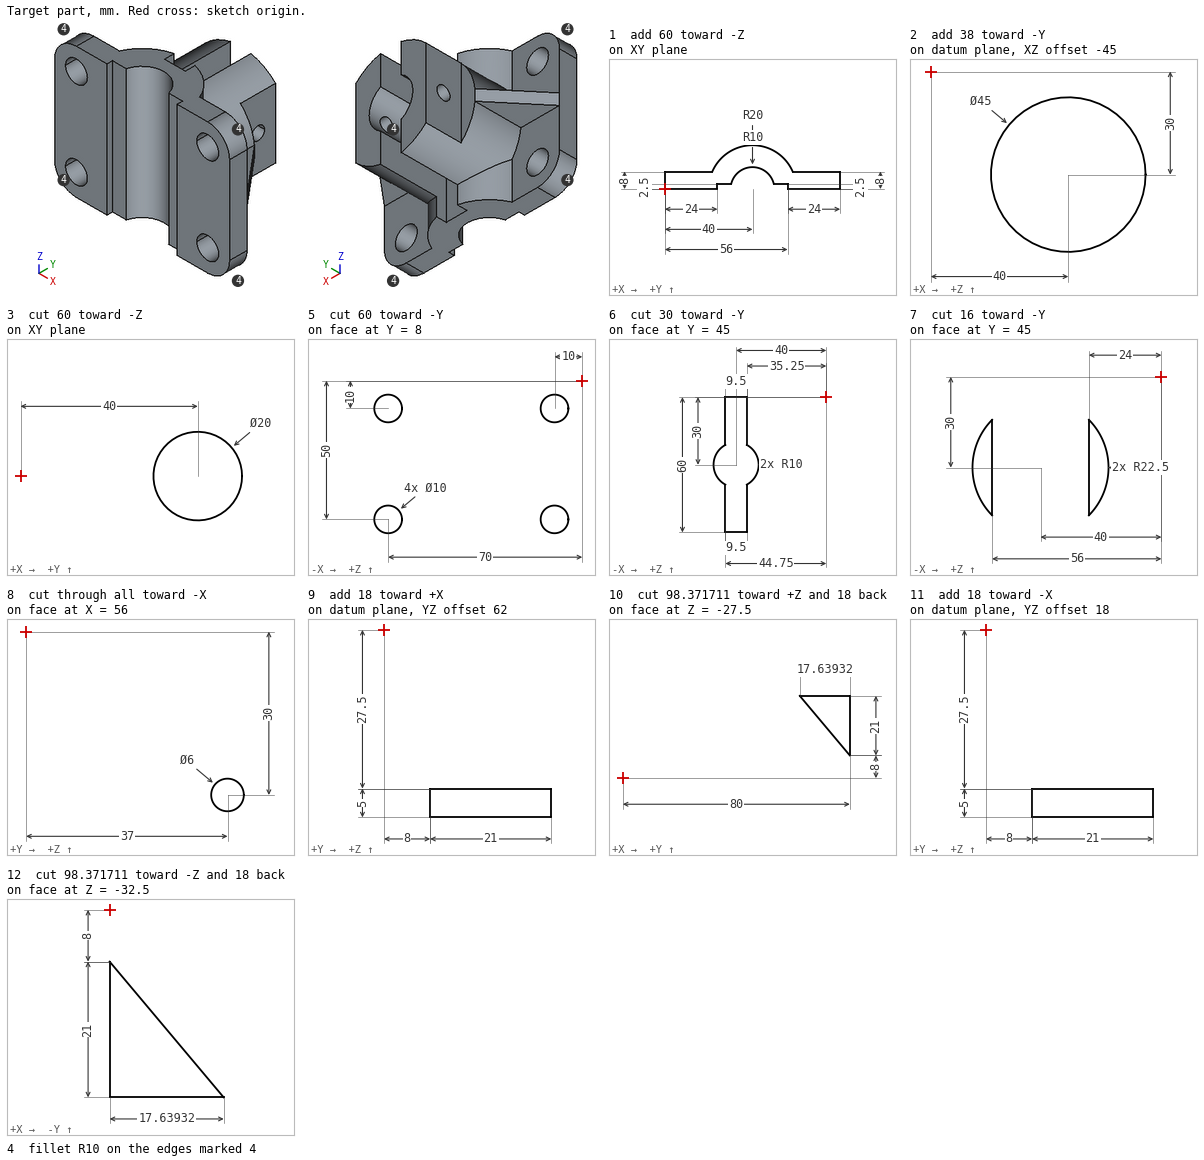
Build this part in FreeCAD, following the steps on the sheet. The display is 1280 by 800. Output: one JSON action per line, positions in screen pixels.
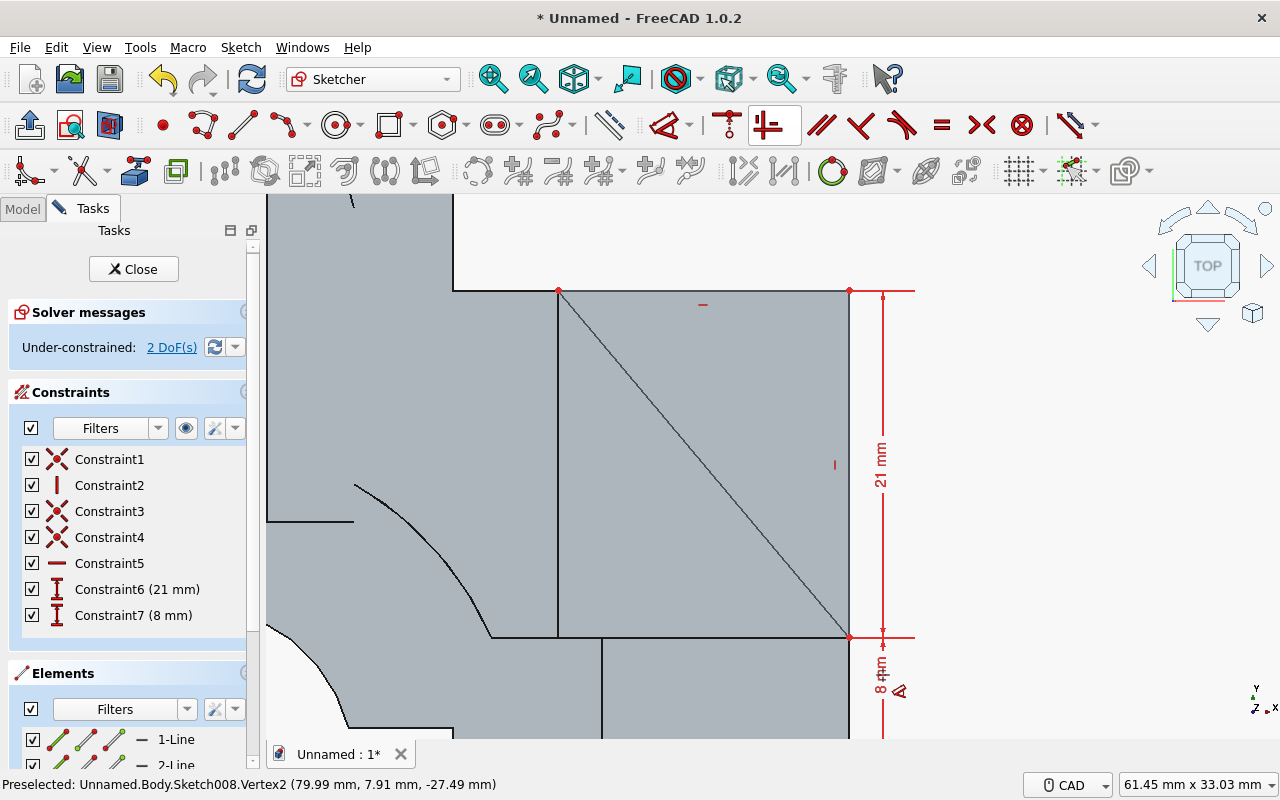
{"action": "left_click", "coordinate": [849, 638]}
{"action": "left_click", "coordinate": [571, 604]}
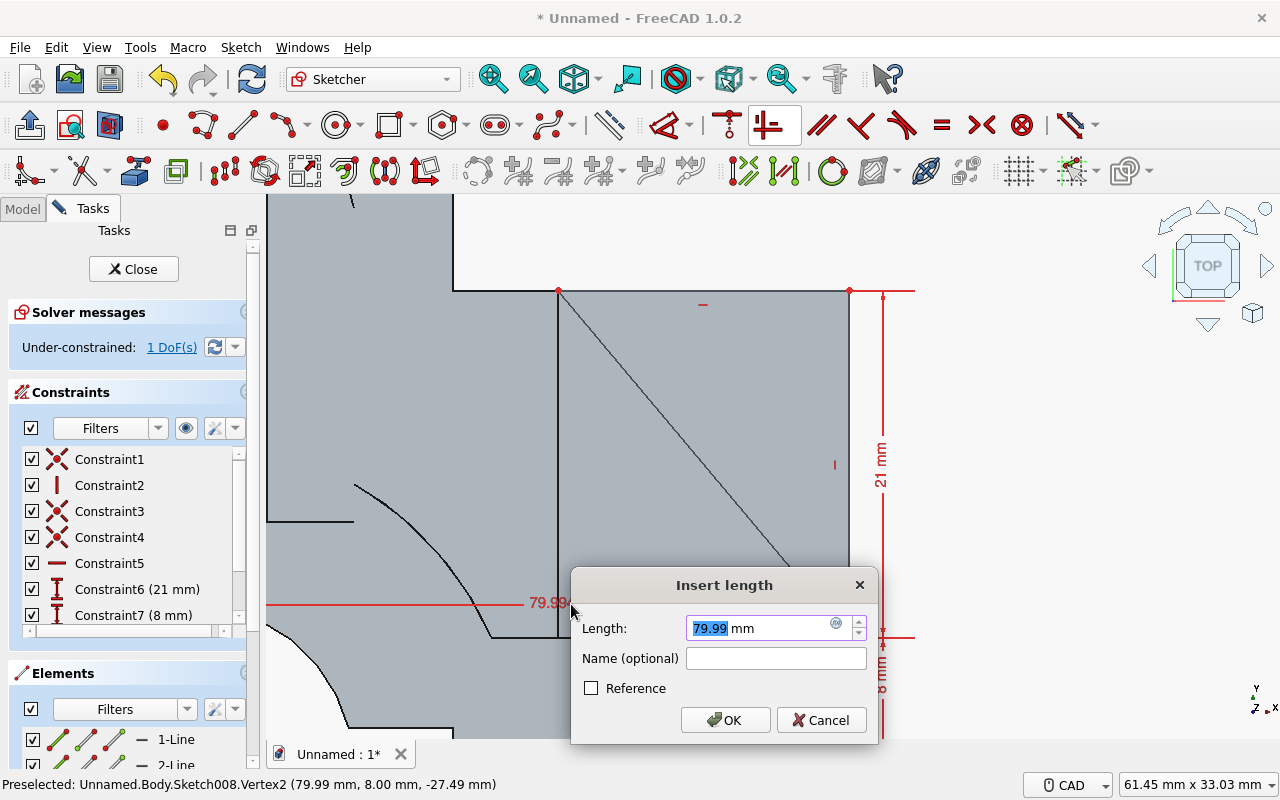
{"action": "type", "text": "80"}
{"action": "key", "text": "Return"}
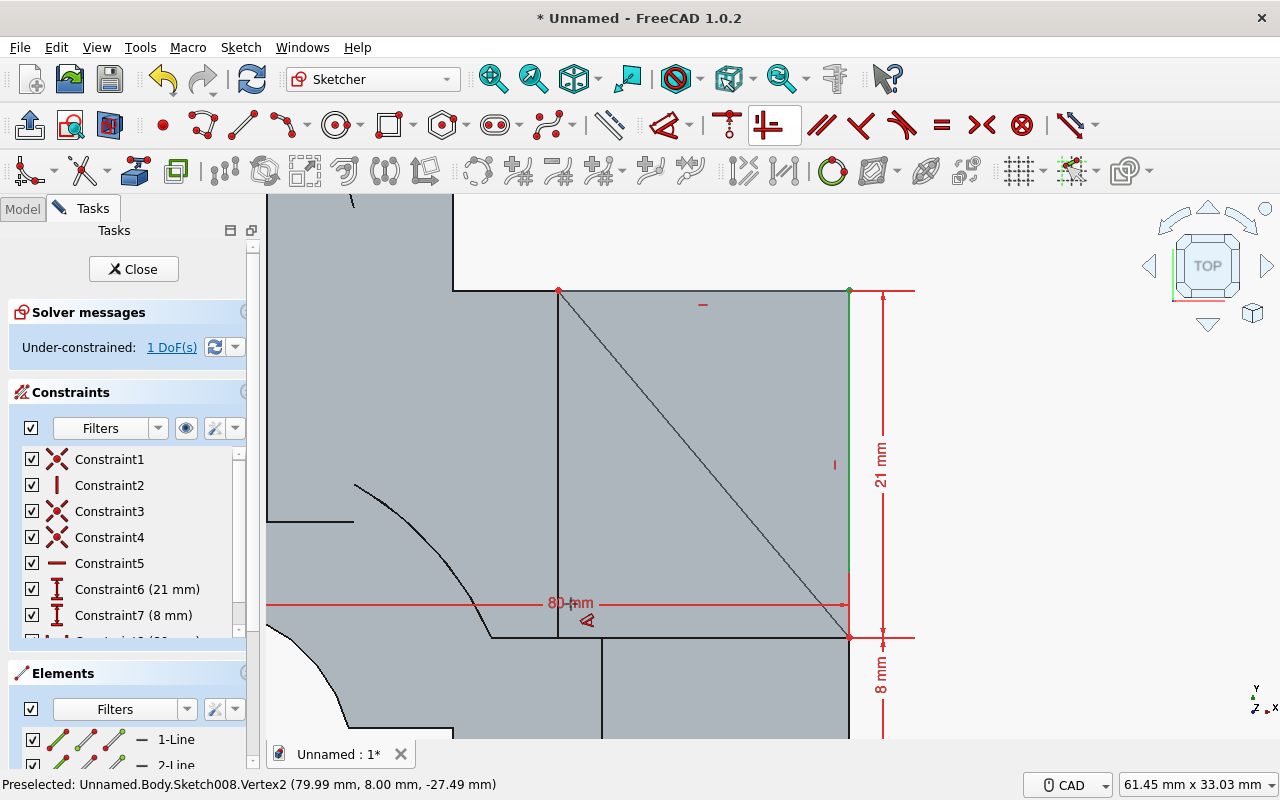
{"action": "left_click", "coordinate": [762, 291]}
{"action": "left_click", "coordinate": [704, 257]}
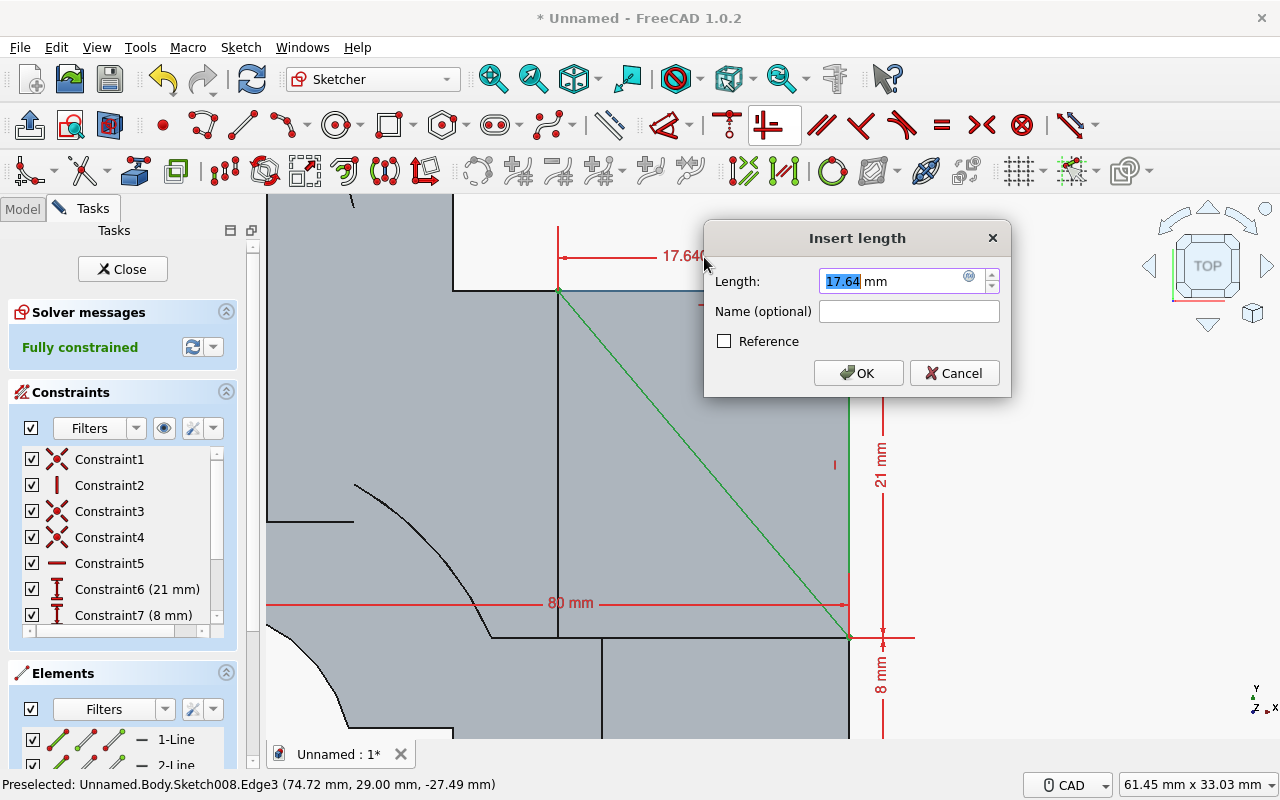
{"action": "type", "text": "17.63932"}
{"action": "key", "text": "Return"}
{"action": "key", "text": "Escape"}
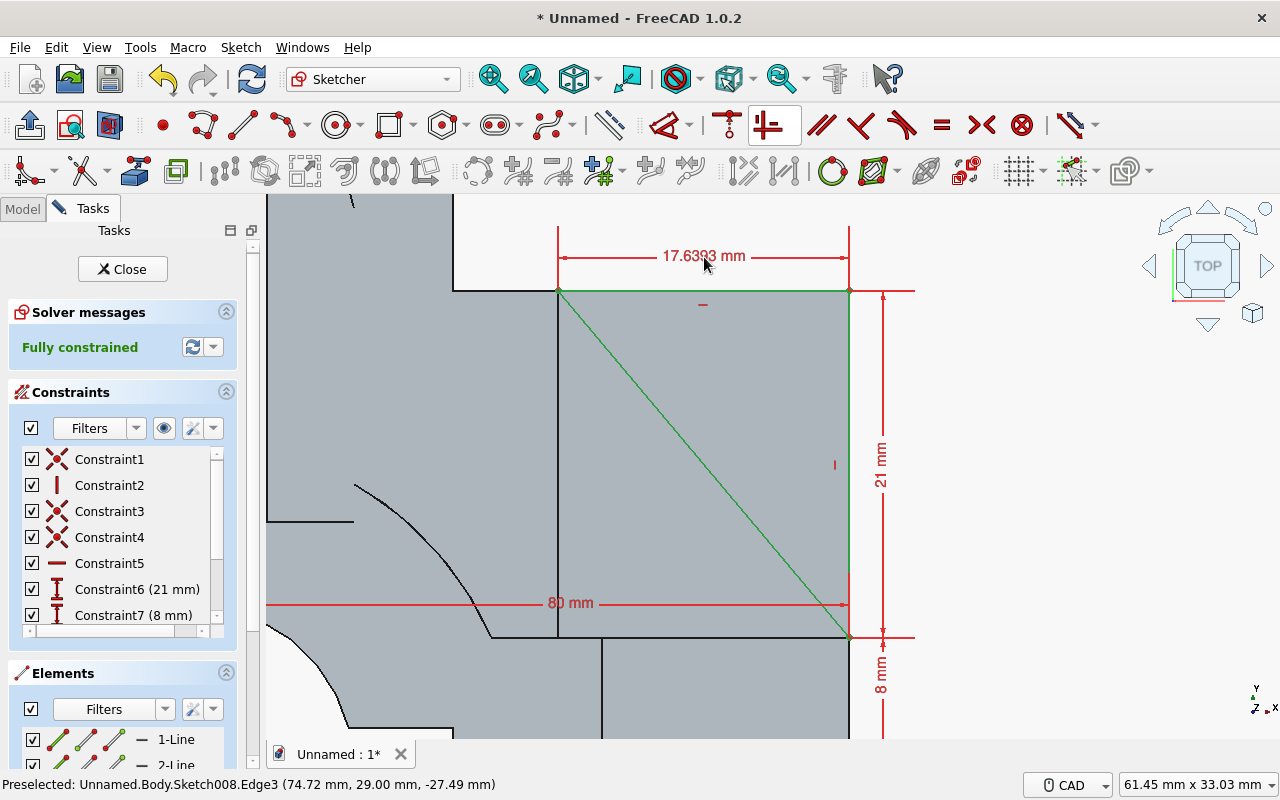
{"action": "left_click", "coordinate": [123, 269]}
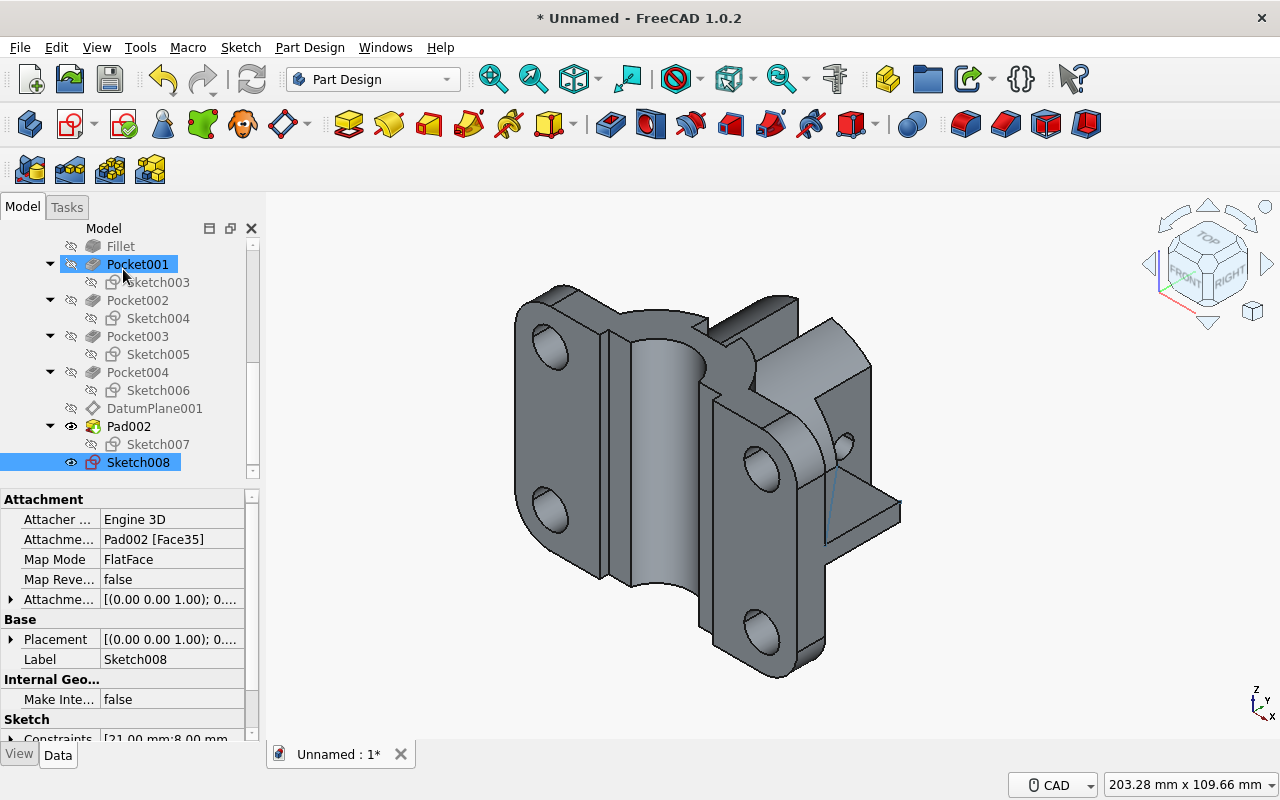
{"action": "left_click", "coordinate": [612, 124]}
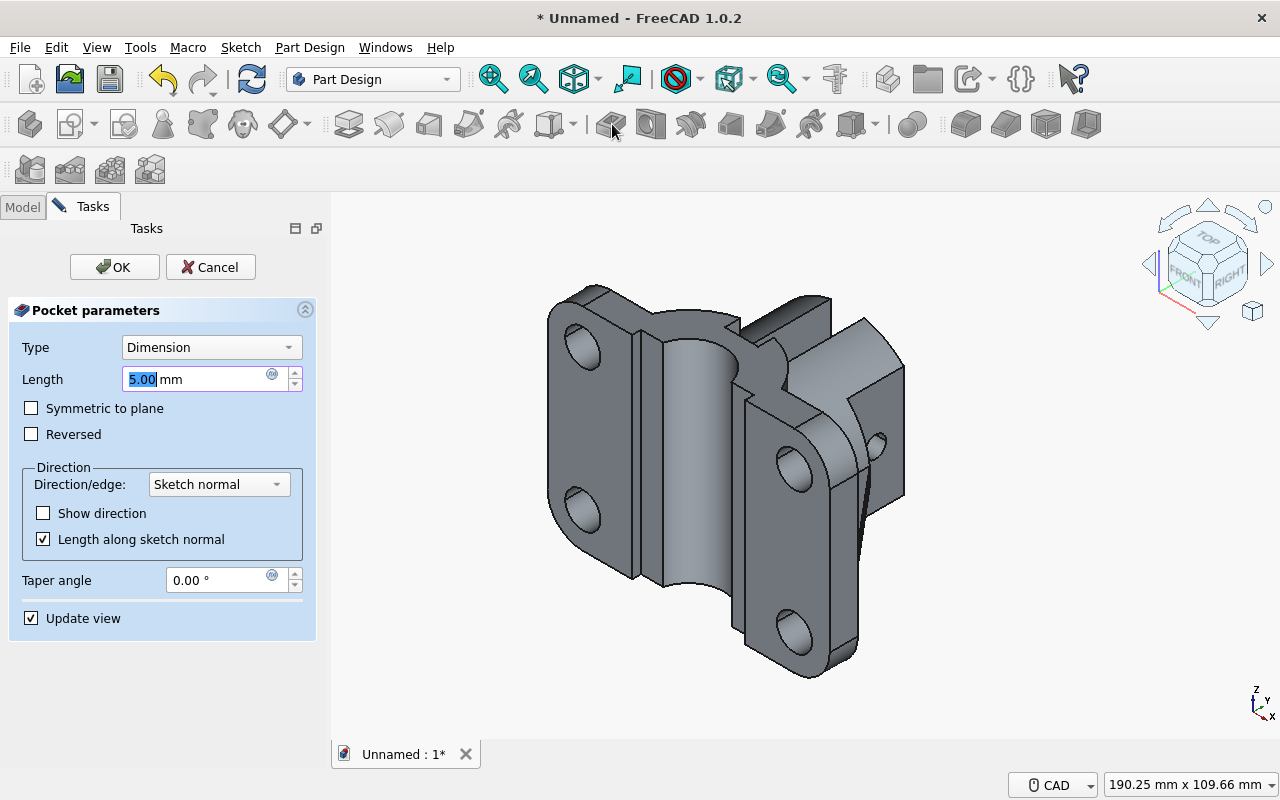
{"action": "left_click", "coordinate": [212, 348]}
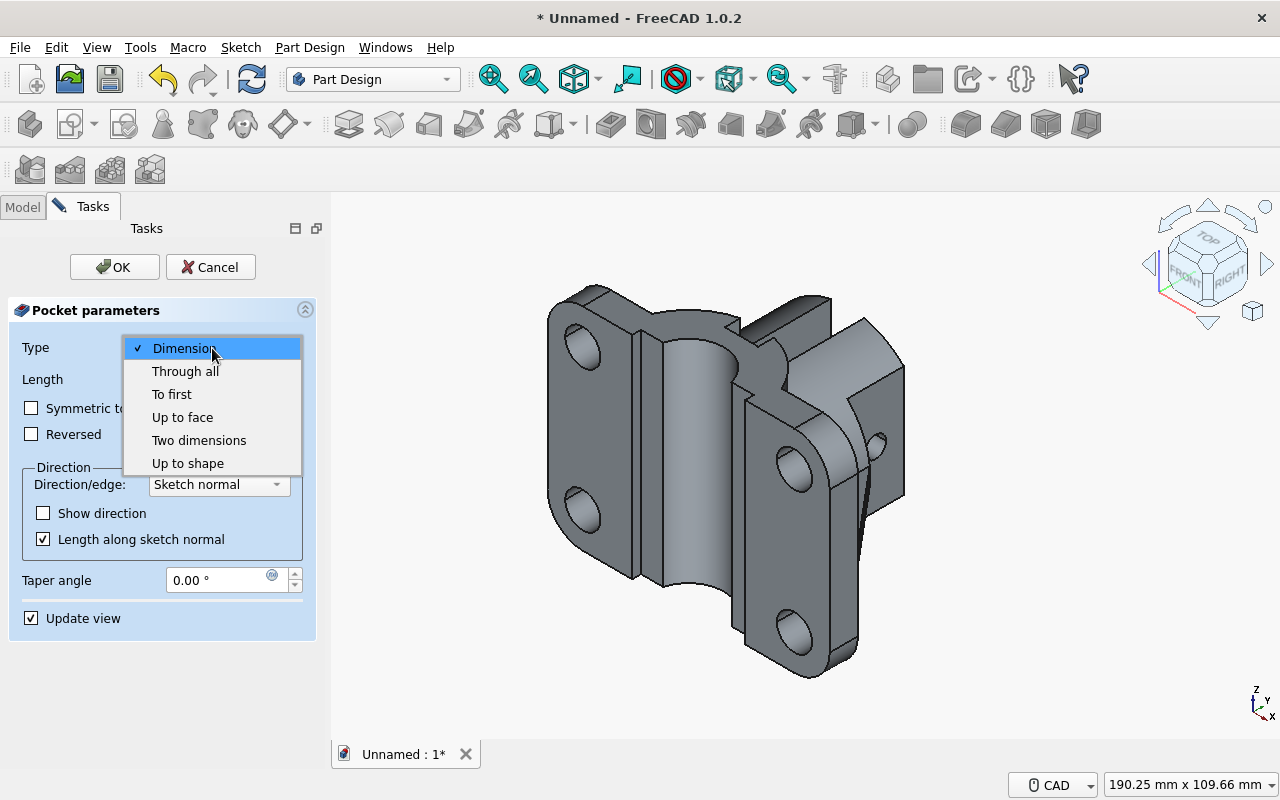
{"action": "left_click", "coordinate": [212, 440]}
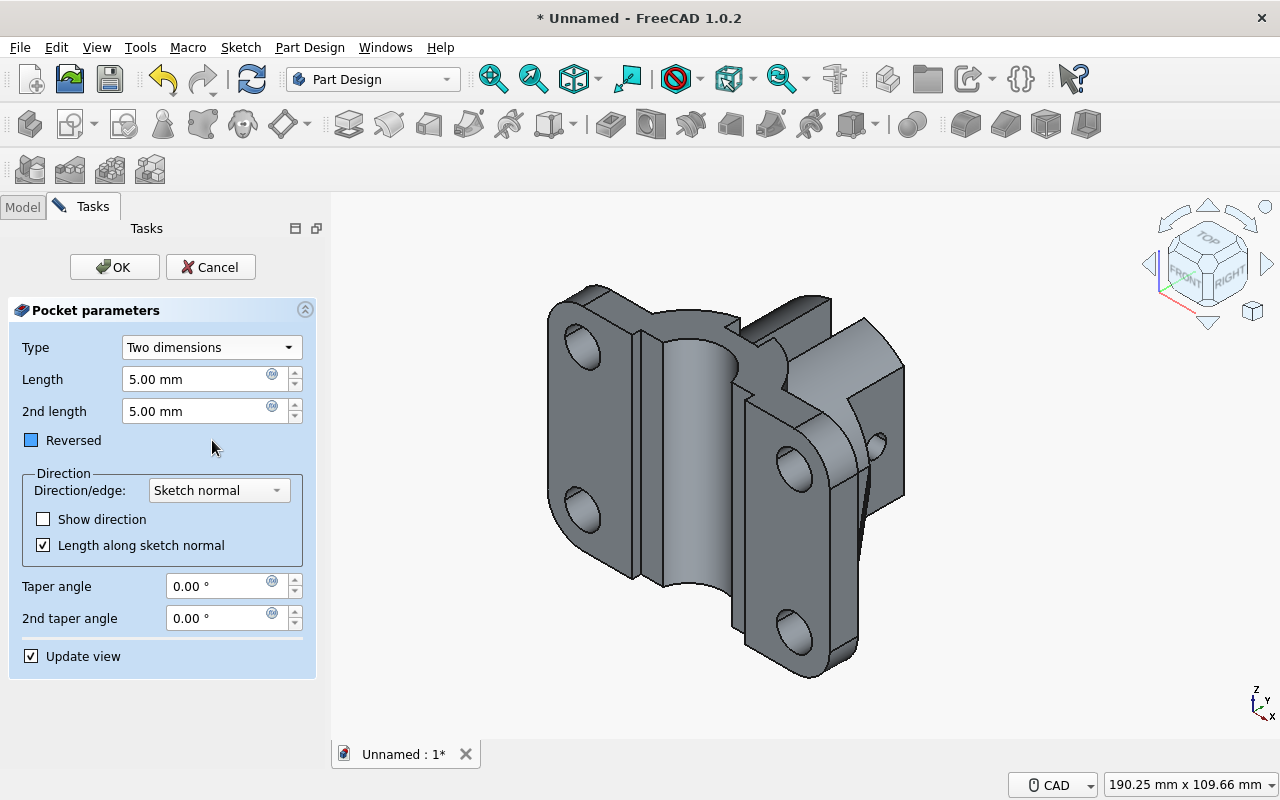
{"action": "triple_click", "coordinate": [204, 379]}